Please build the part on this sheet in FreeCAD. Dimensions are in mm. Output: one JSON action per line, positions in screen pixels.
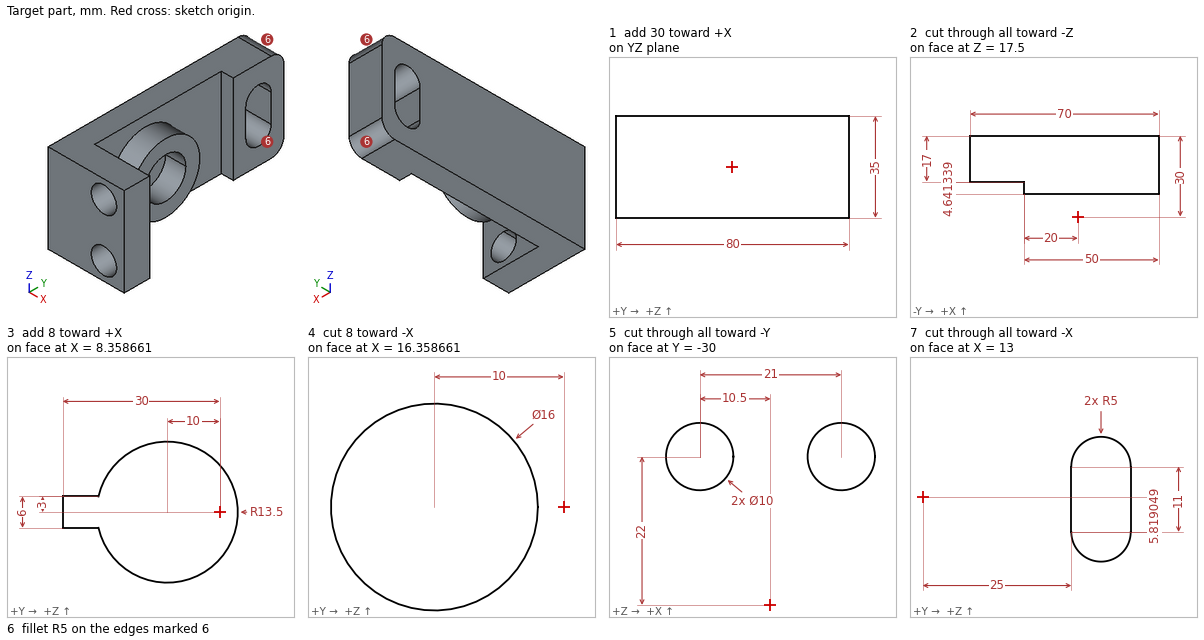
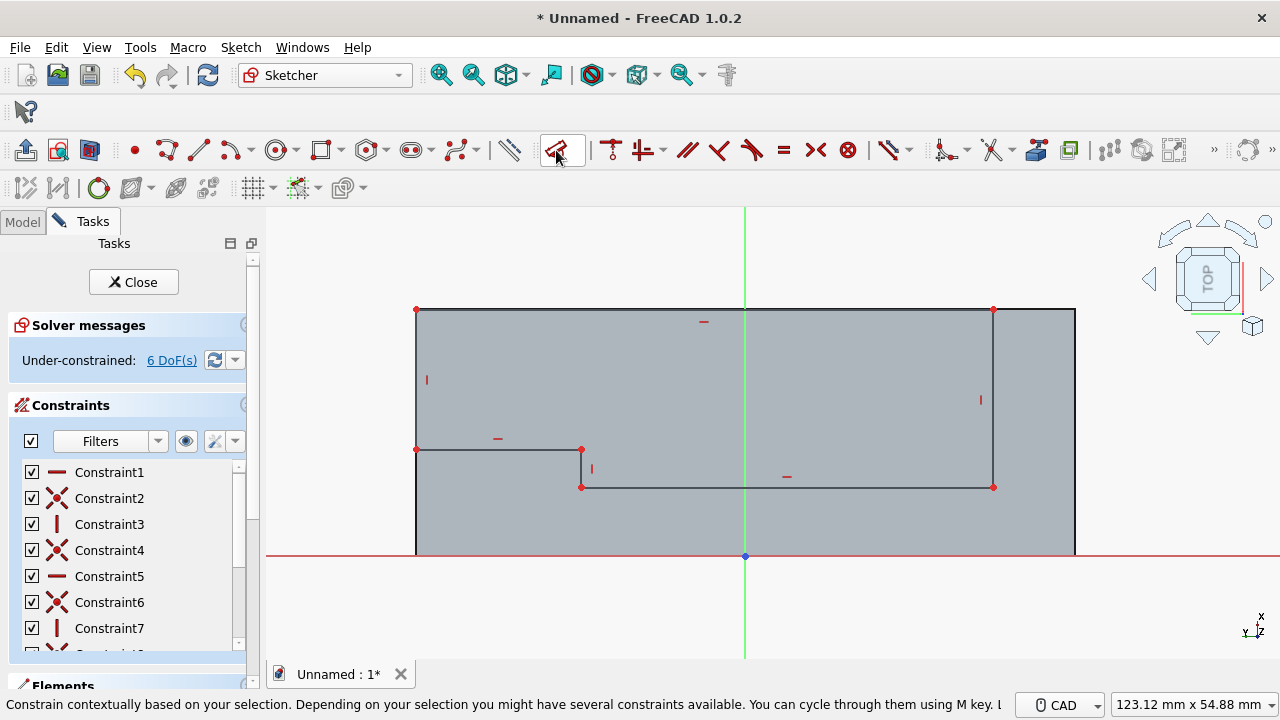
{"action": "left_click", "coordinate": [705, 488]}
{"action": "left_click", "coordinate": [787, 522]}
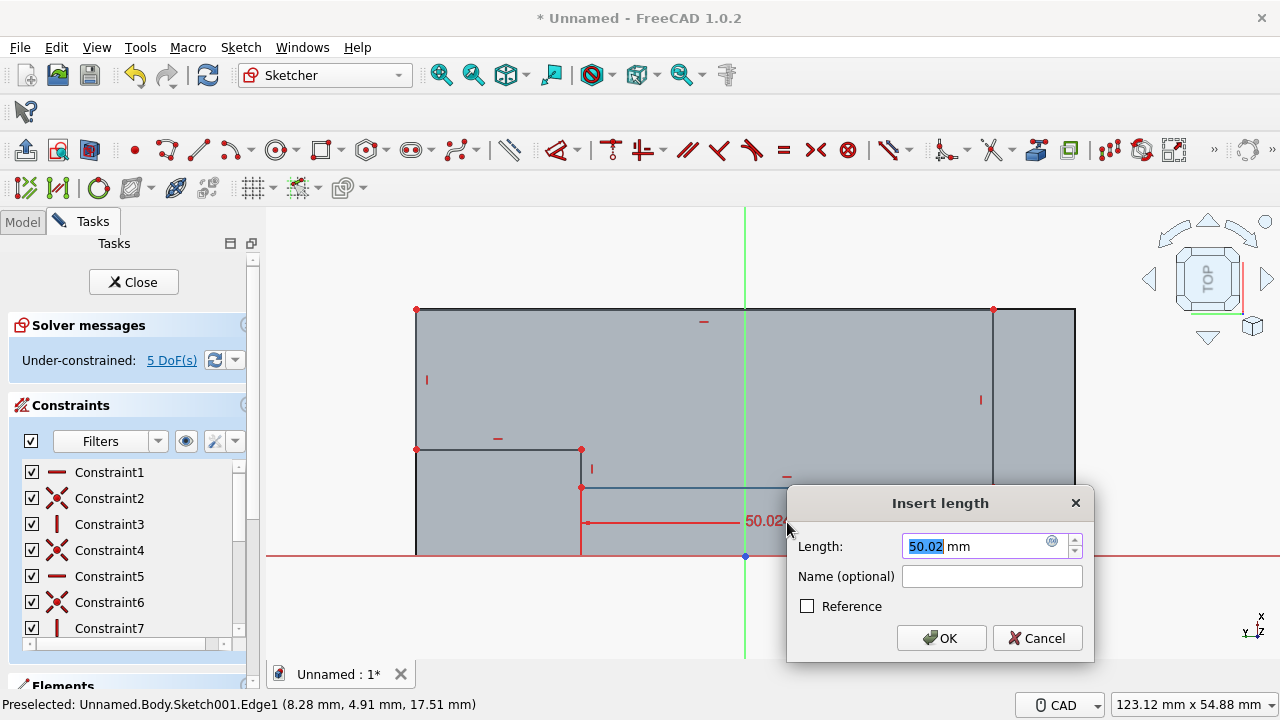
{"action": "type", "text": "50"}
{"action": "key", "text": "Return"}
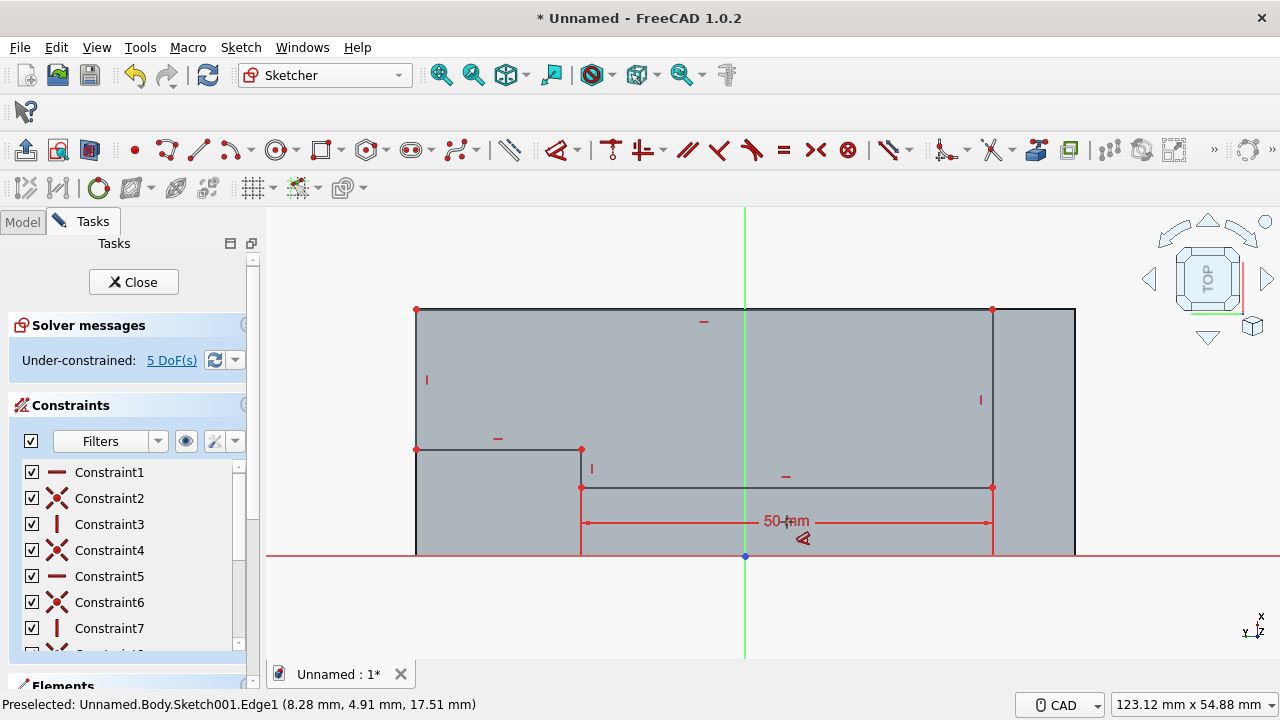
{"action": "left_click", "coordinate": [820, 310]}
{"action": "left_click", "coordinate": [704, 276]}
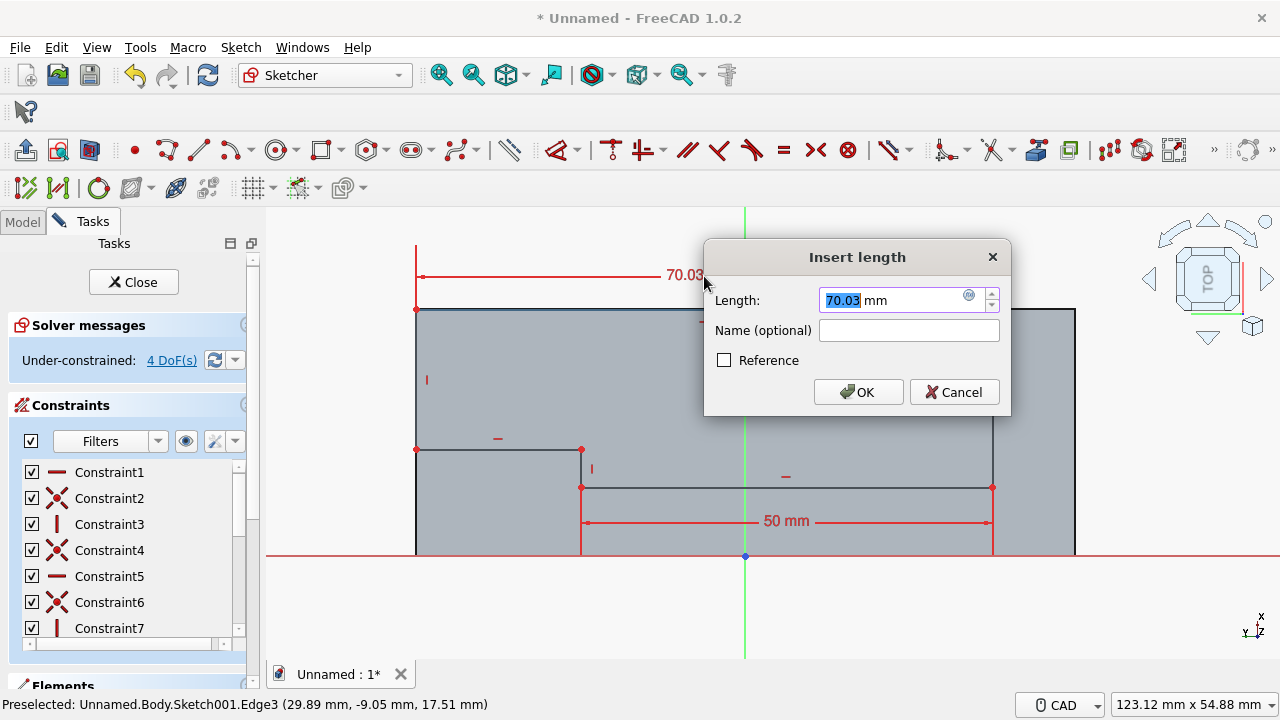
{"action": "type", "text": "70"}
{"action": "key", "text": "Return"}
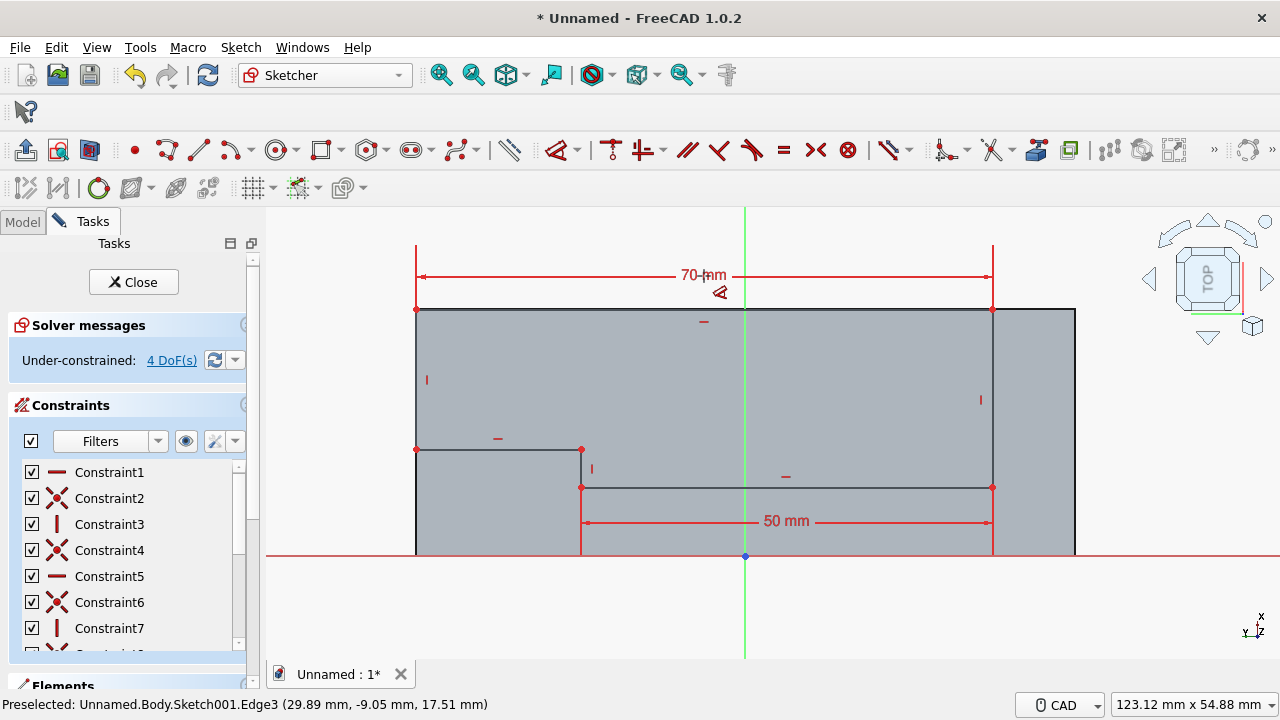
{"action": "left_click", "coordinate": [416, 352]}
{"action": "left_click", "coordinate": [382, 380]}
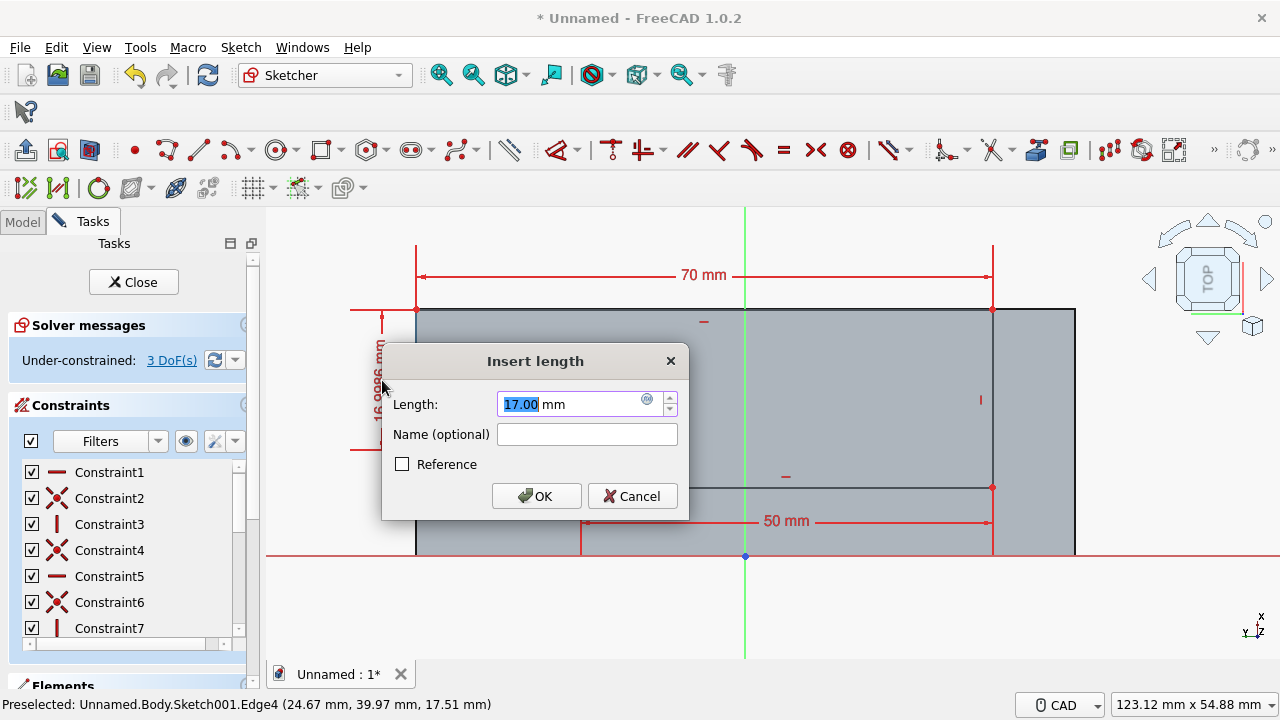
{"action": "type", "text": "17"}
{"action": "key", "text": "Return"}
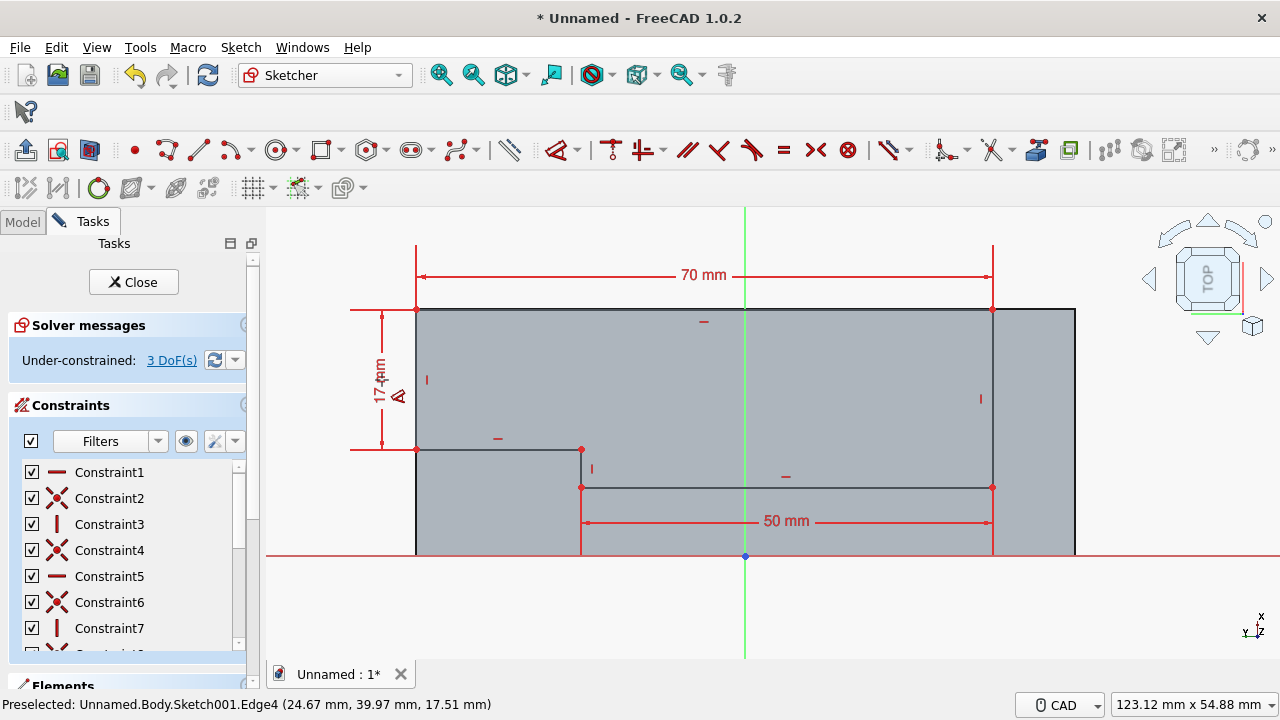
{"action": "left_click", "coordinate": [581, 488]}
{"action": "left_click", "coordinate": [663, 590]}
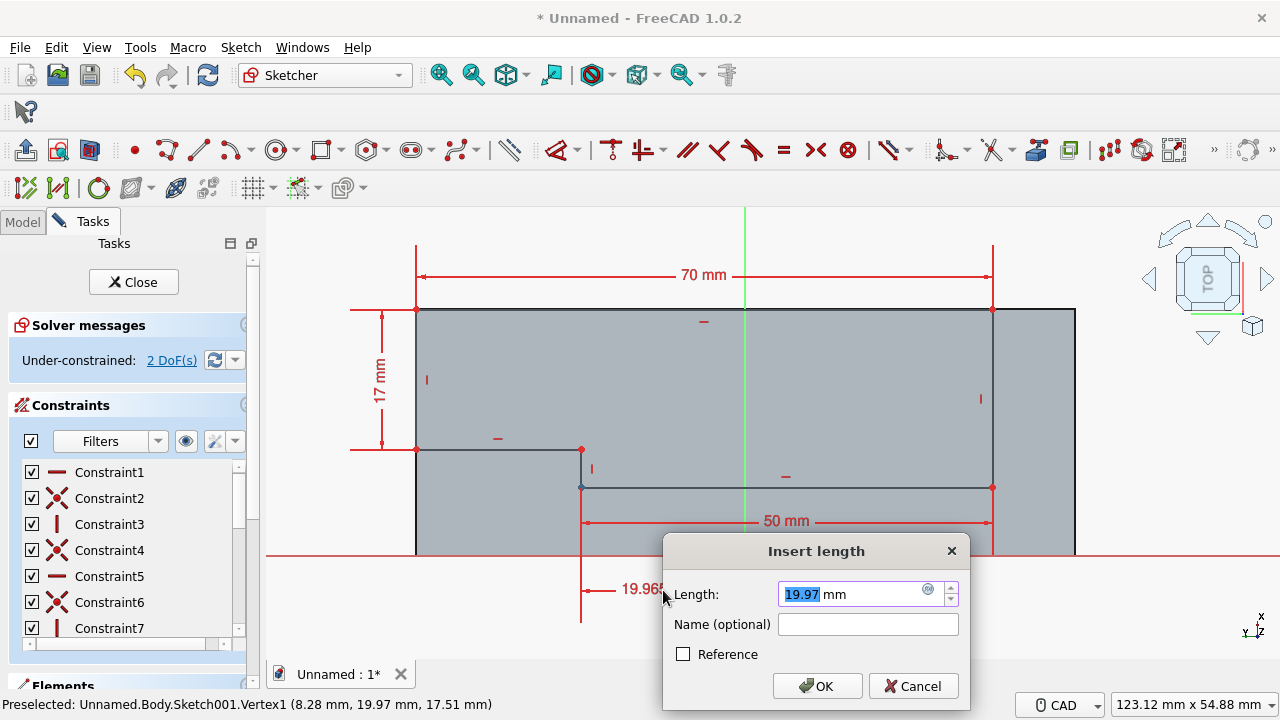
{"action": "type", "text": "20"}
{"action": "key", "text": "Return"}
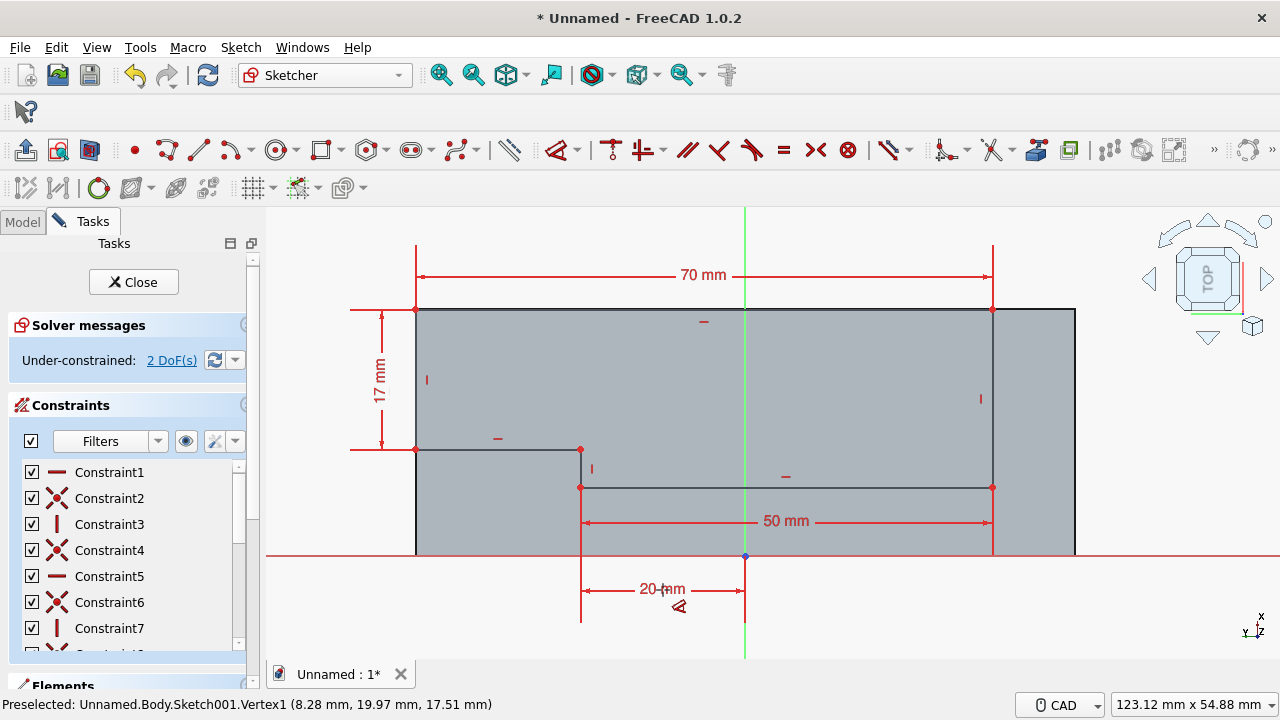
{"action": "left_click", "coordinate": [993, 310]}
{"action": "left_click", "coordinate": [1027, 433]}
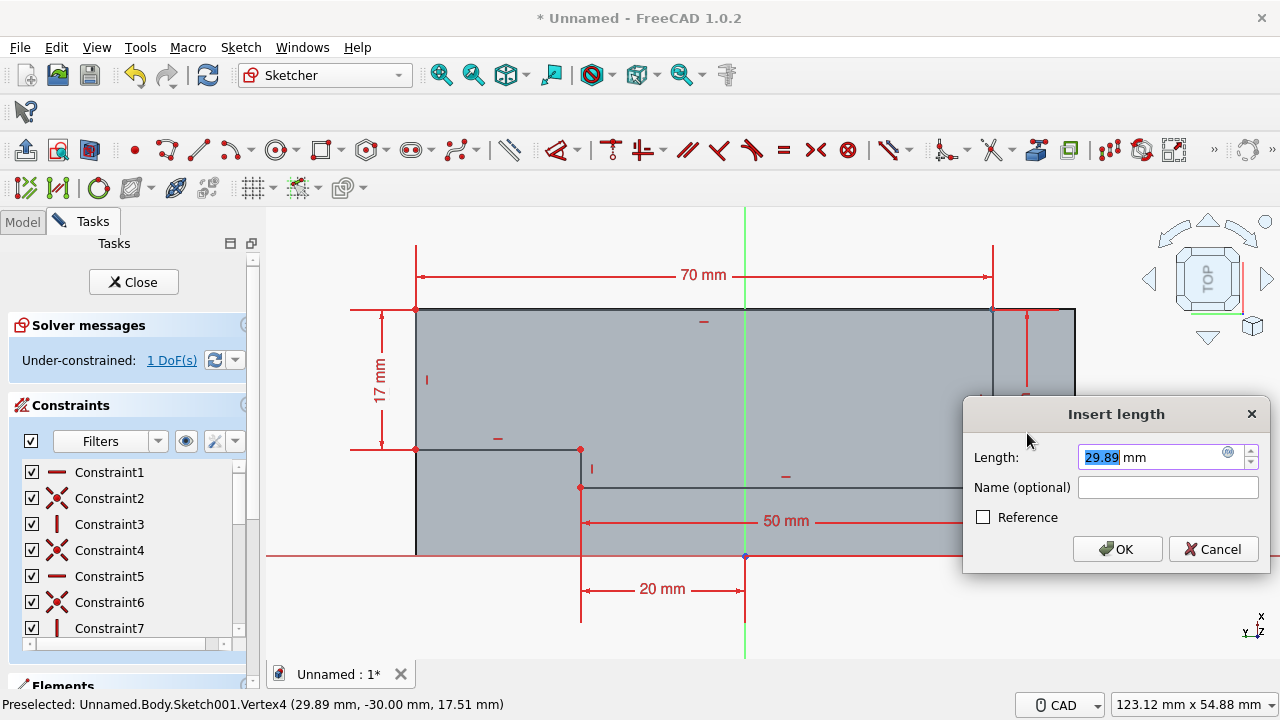
{"action": "type", "text": "30"}
{"action": "key", "text": "Return"}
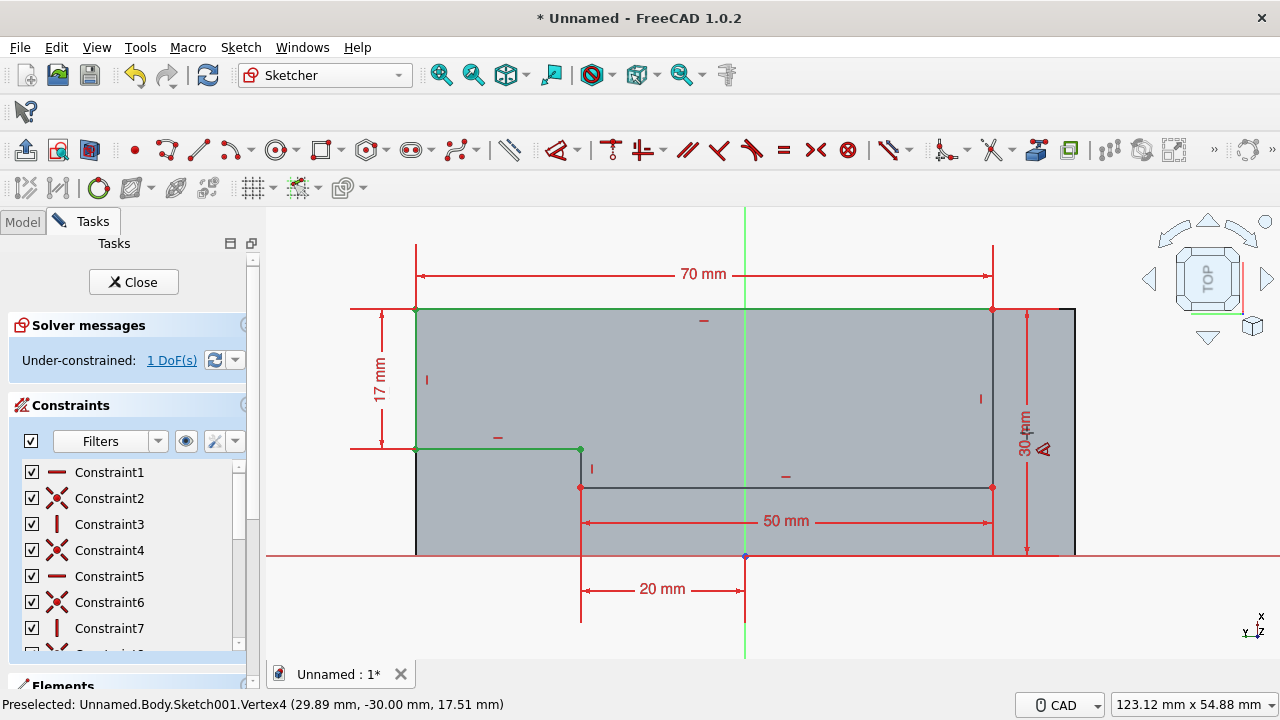
{"action": "left_click", "coordinate": [581, 461]}
{"action": "left_click", "coordinate": [547, 469]}